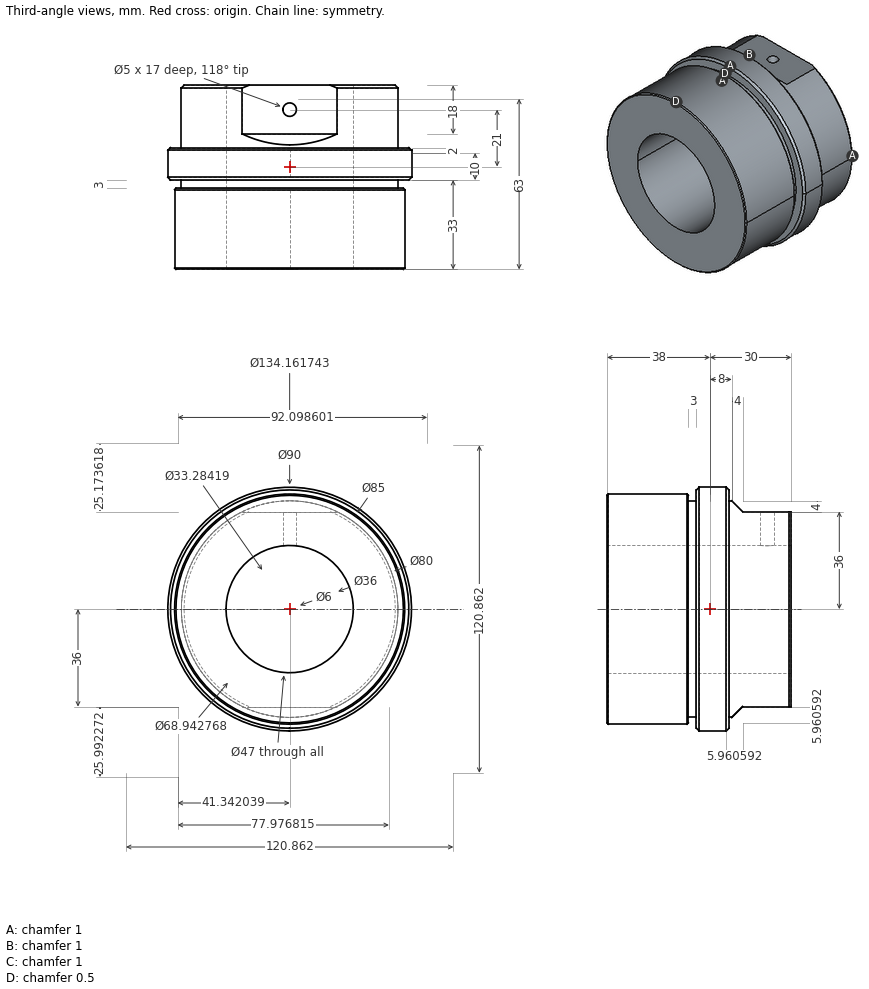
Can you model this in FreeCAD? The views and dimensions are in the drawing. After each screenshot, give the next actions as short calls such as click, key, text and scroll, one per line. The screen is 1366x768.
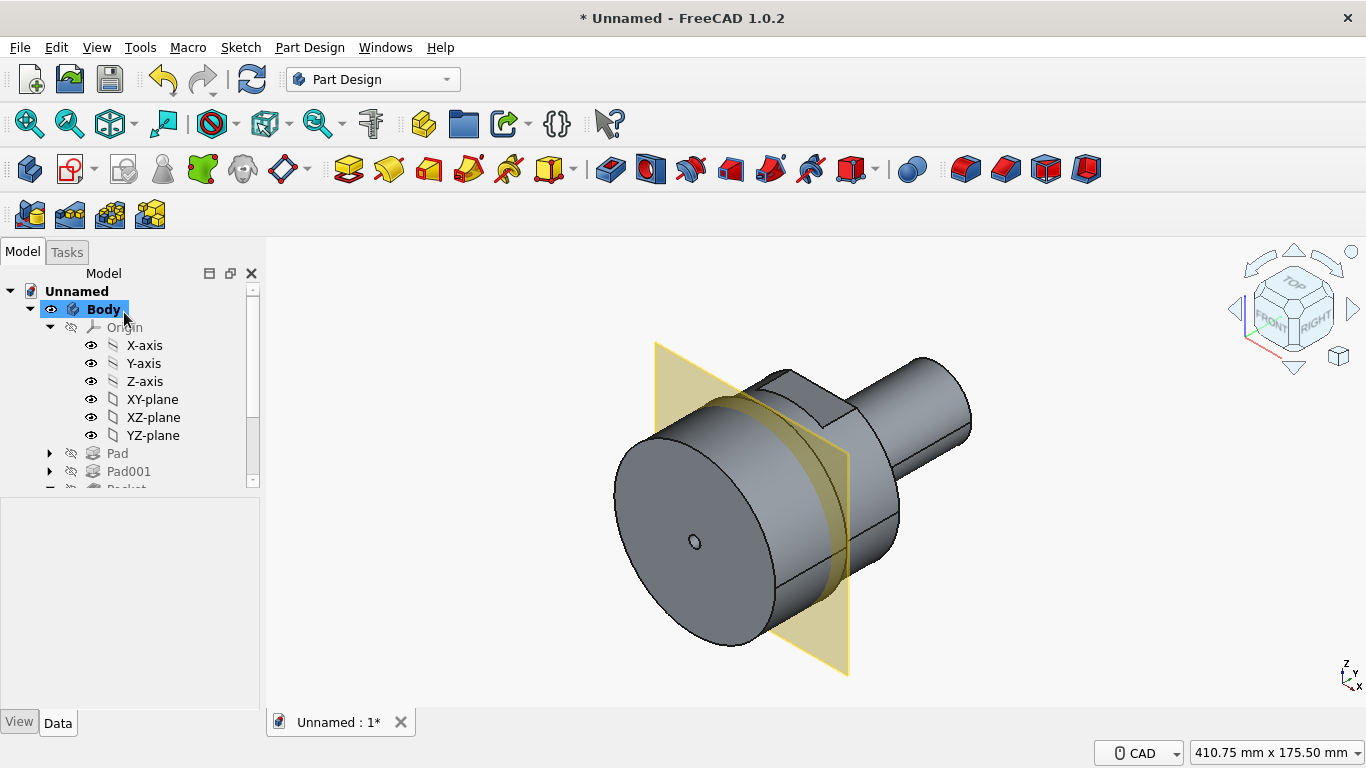
scroll(100, 377, down, 3)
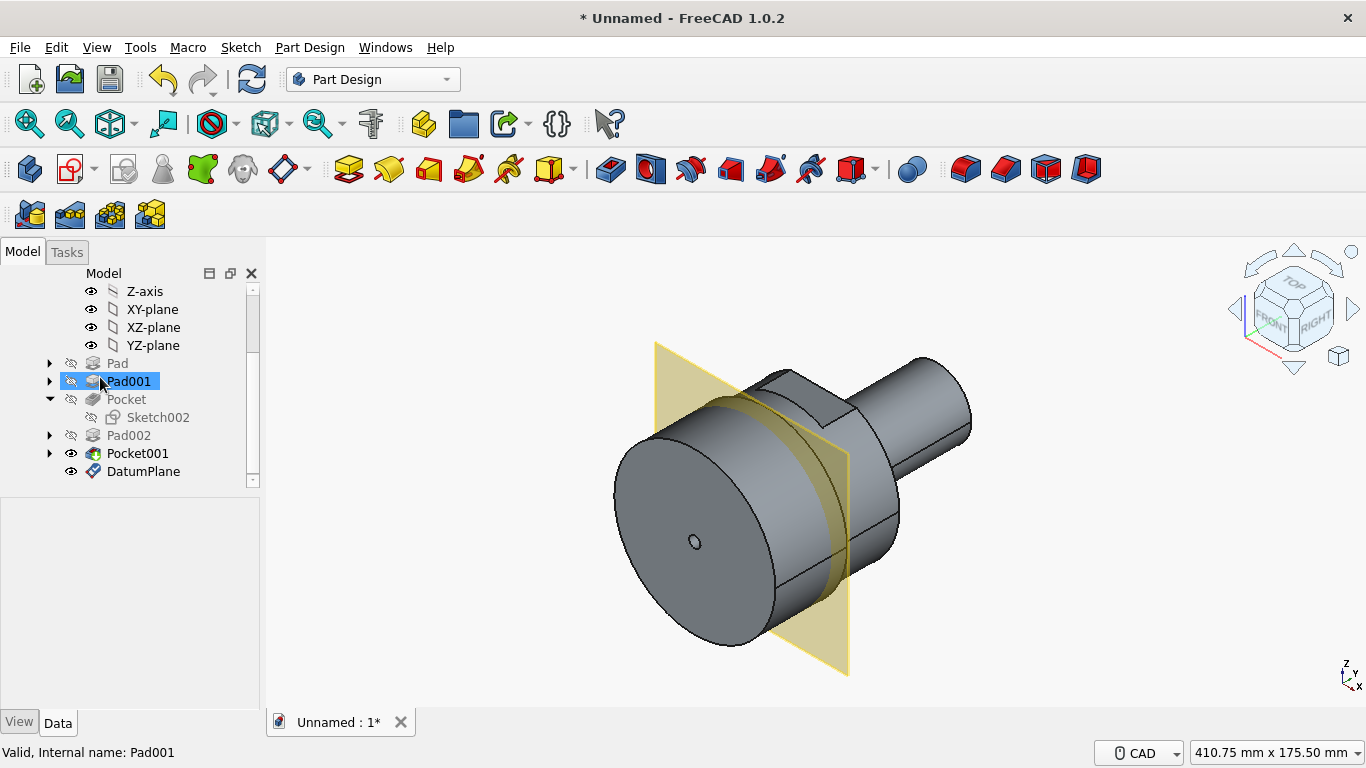
click(116, 471)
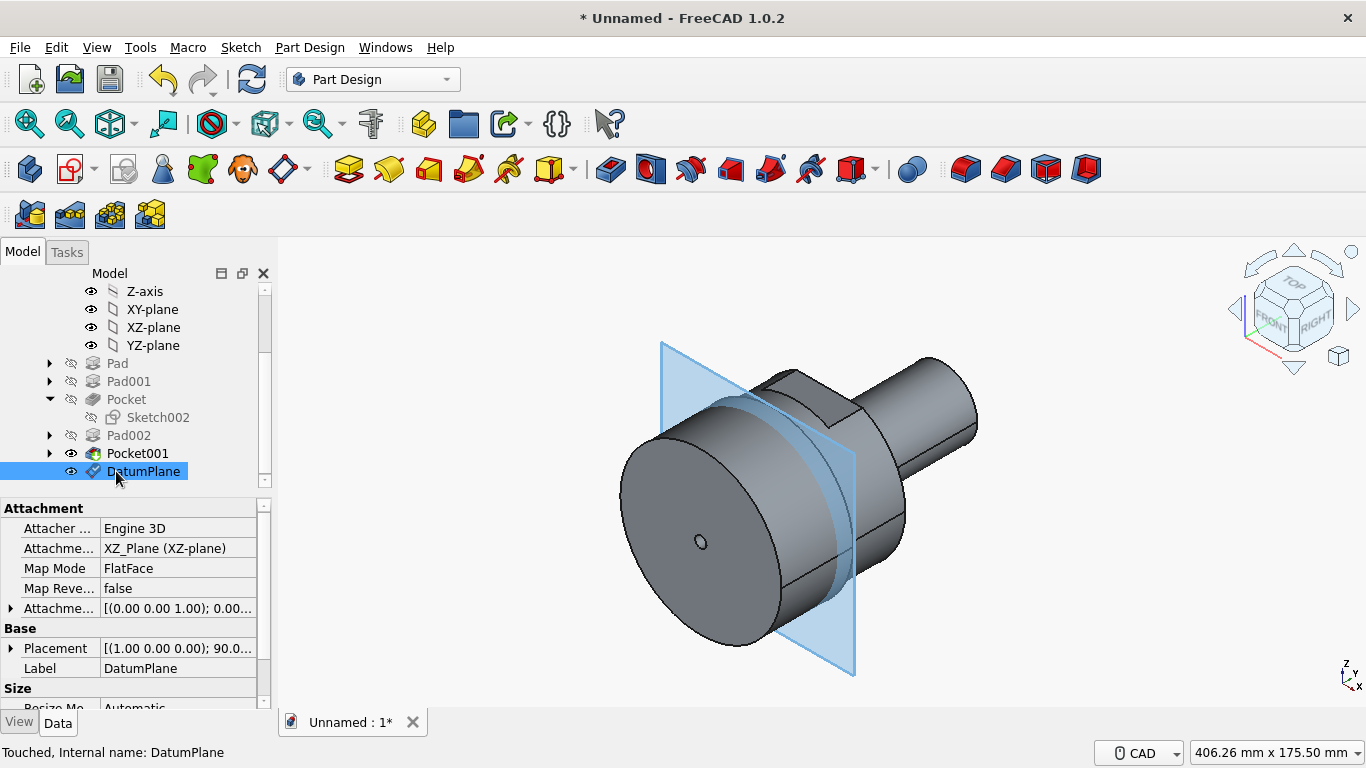
click(70, 170)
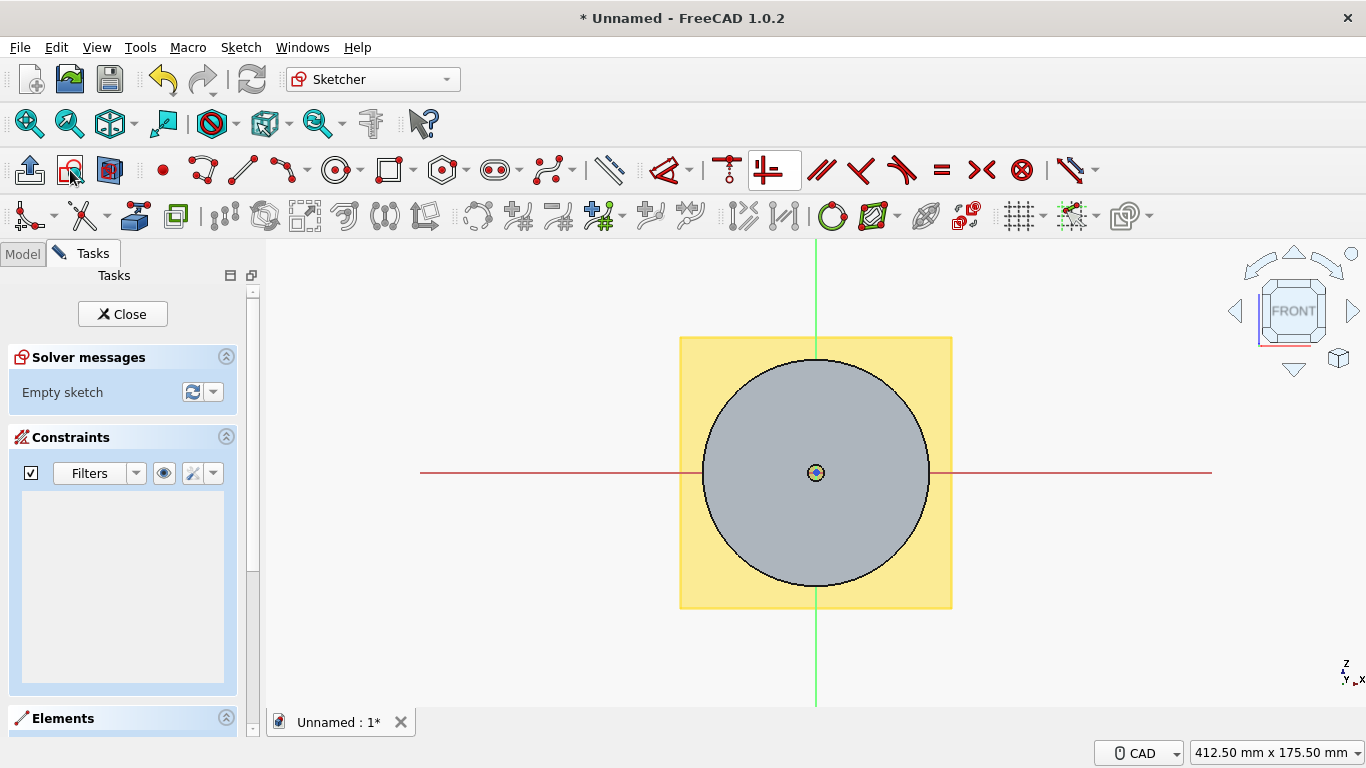
click(110, 170)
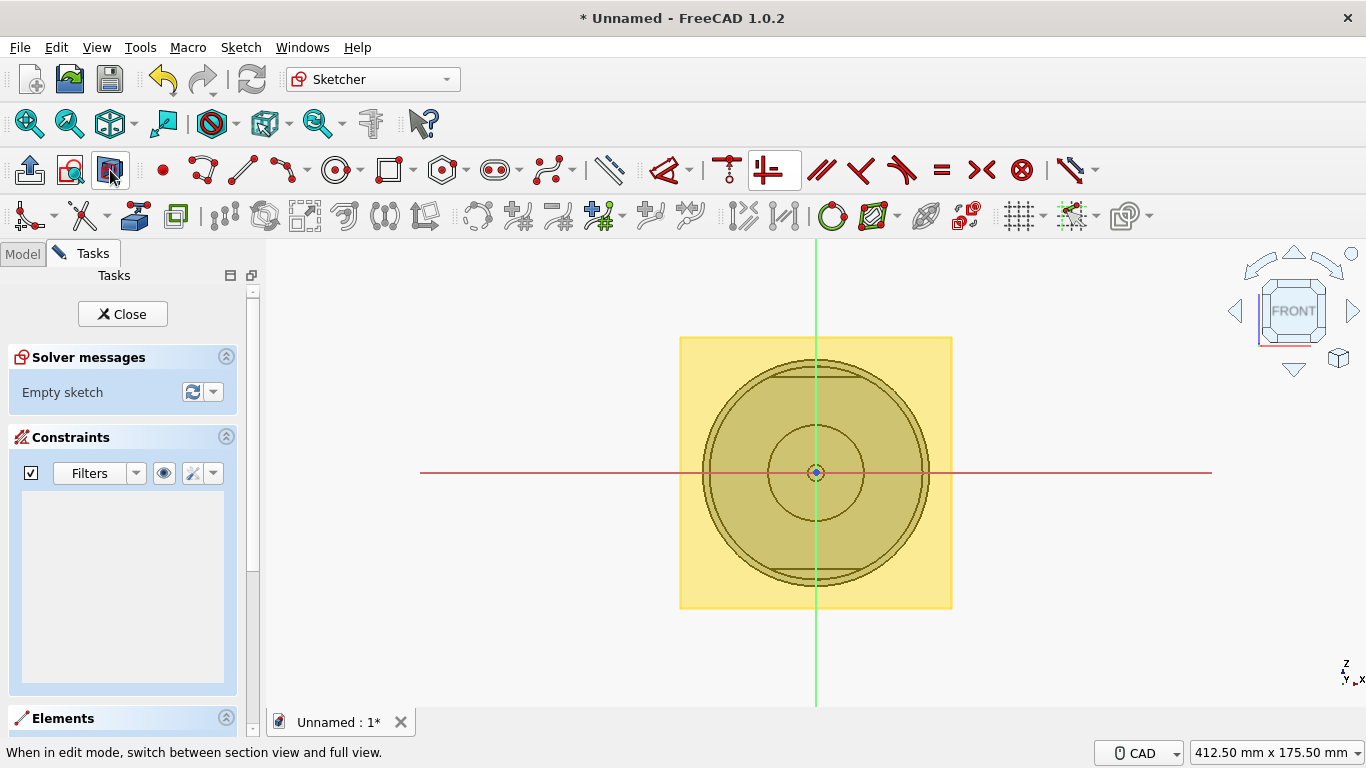
click(336, 170)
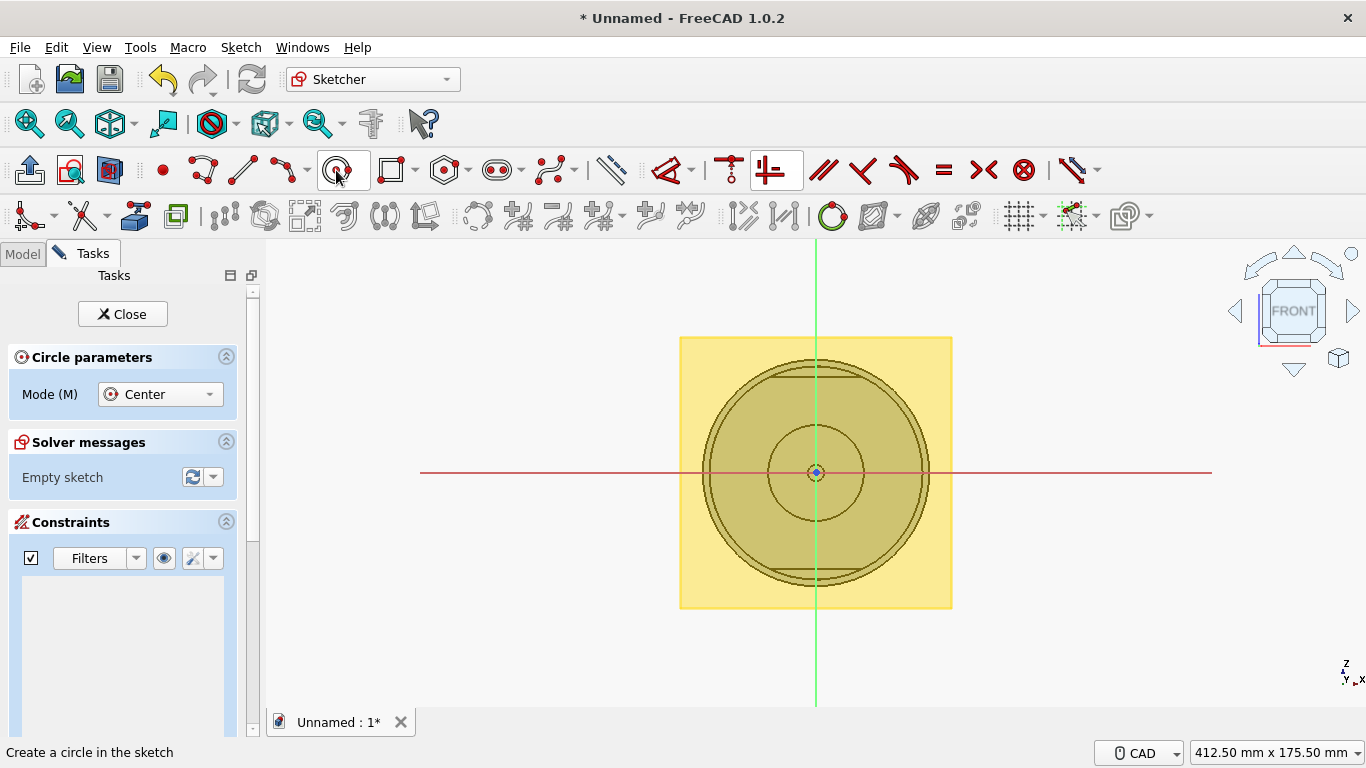
click(816, 473)
click(942, 347)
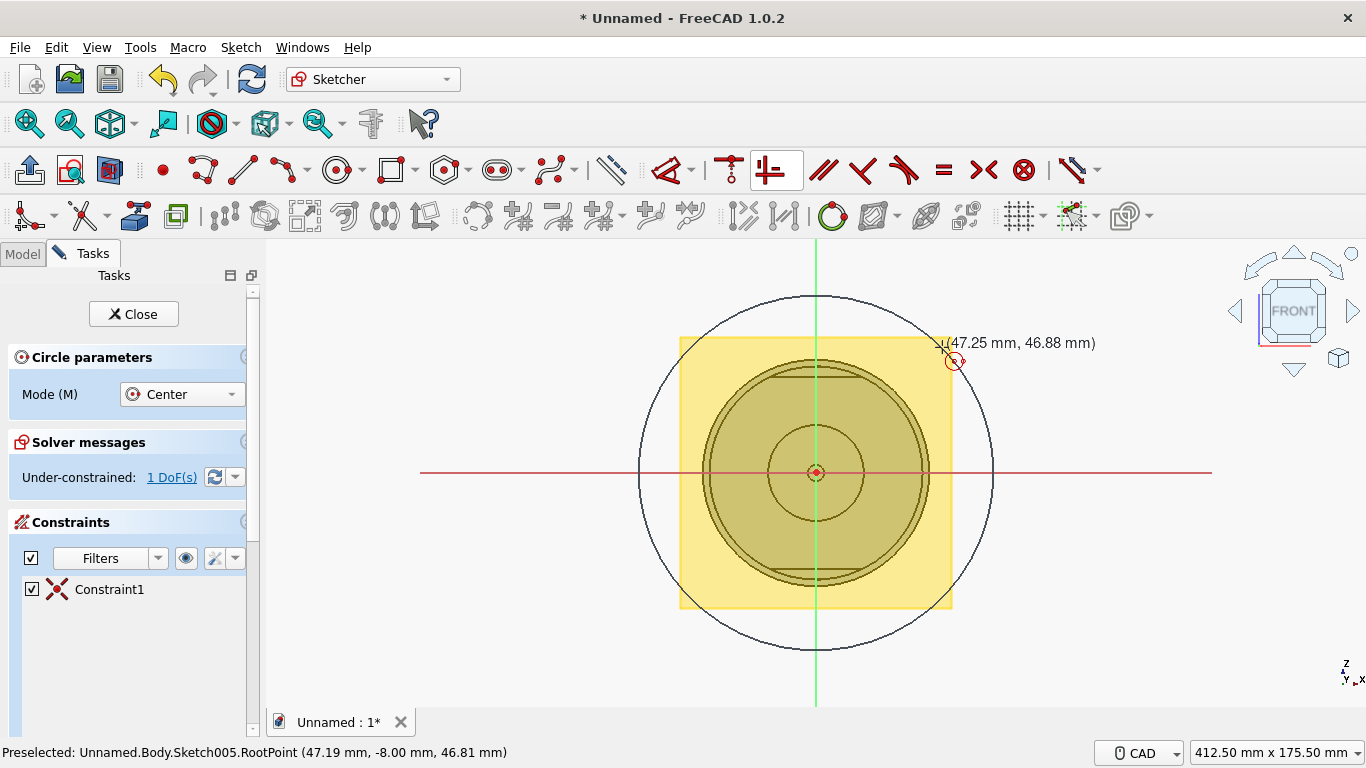
click(816, 473)
click(891, 398)
key(Escape)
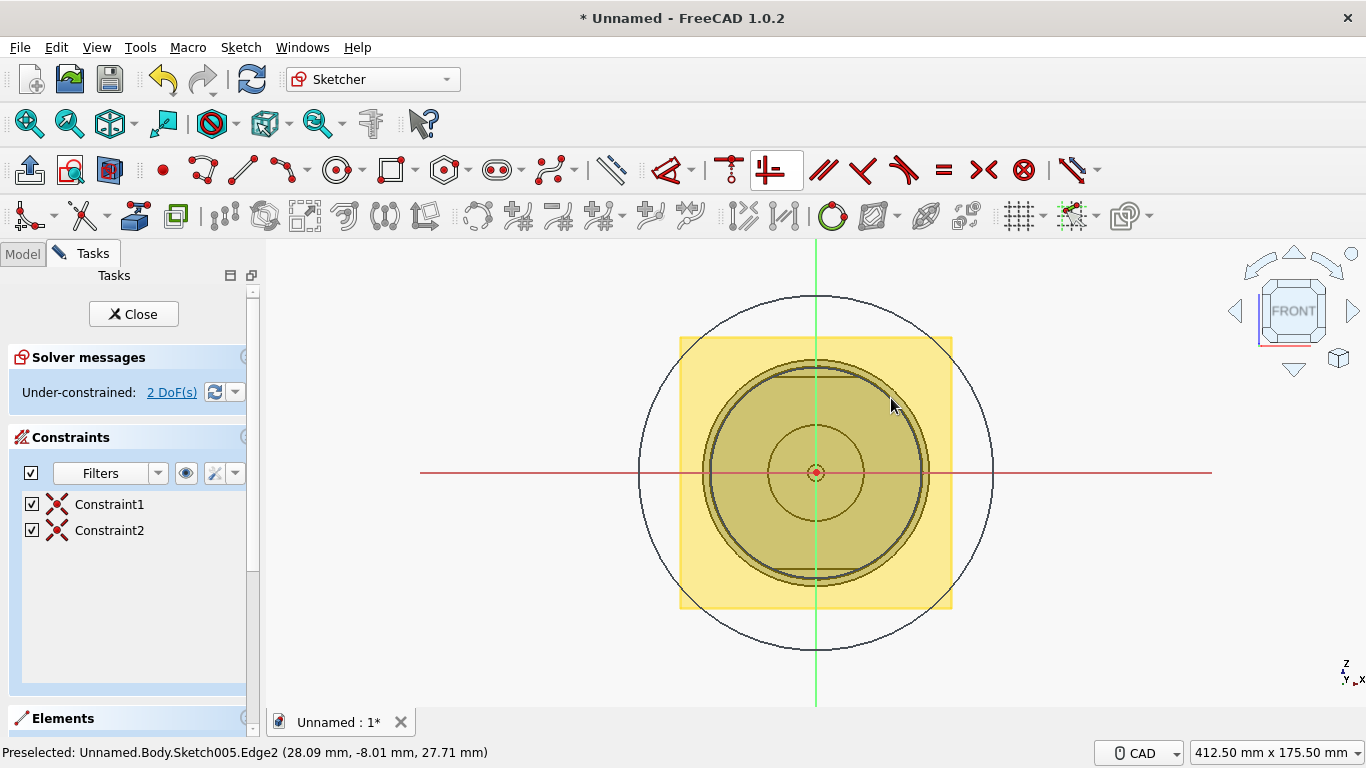
click(666, 170)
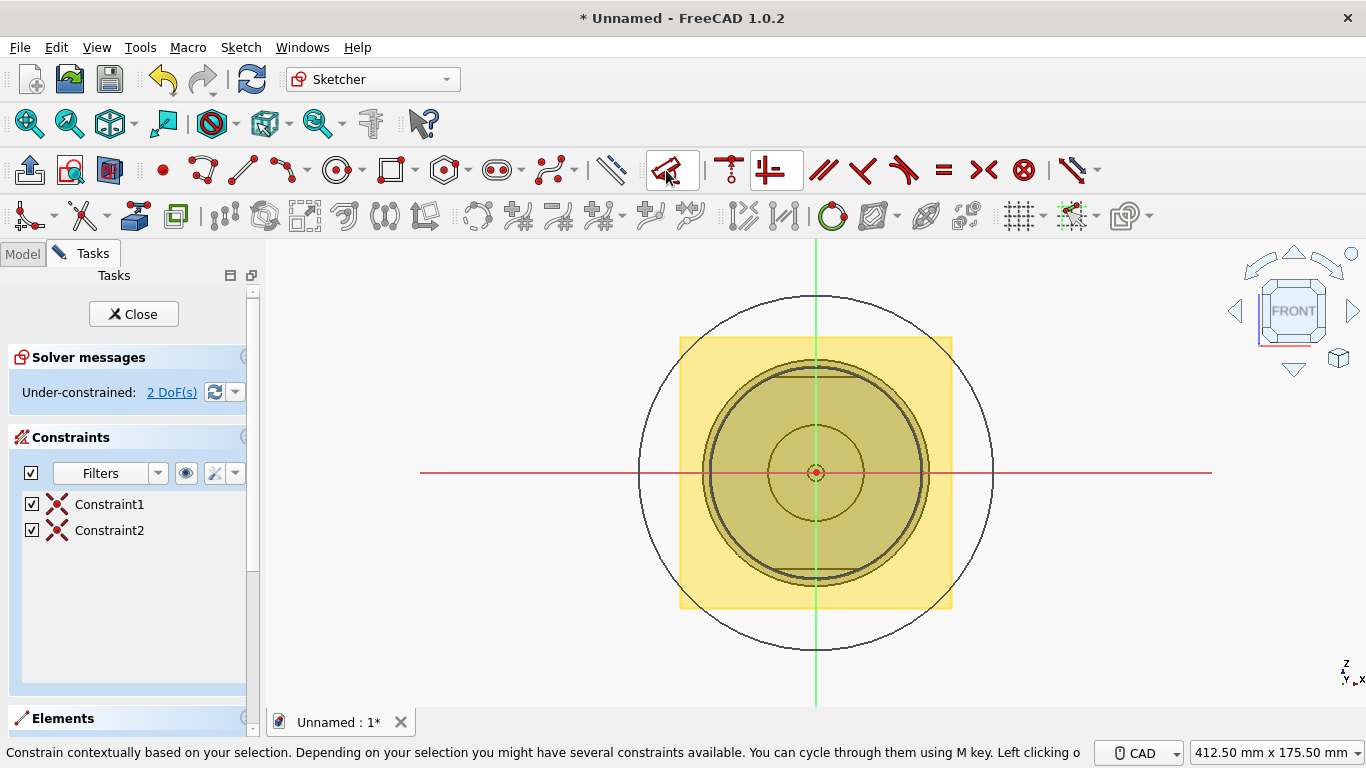
click(941, 347)
click(964, 324)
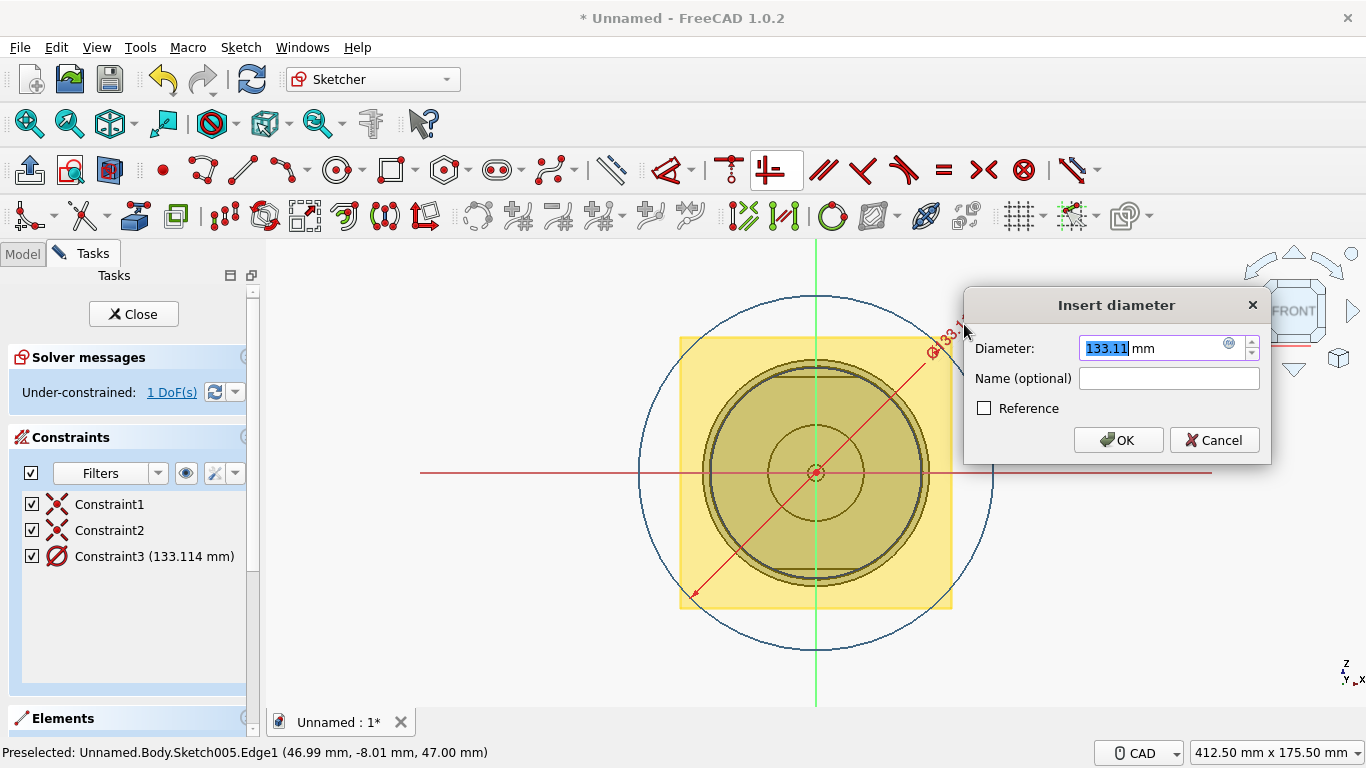
text(134.161743)
key(Return)